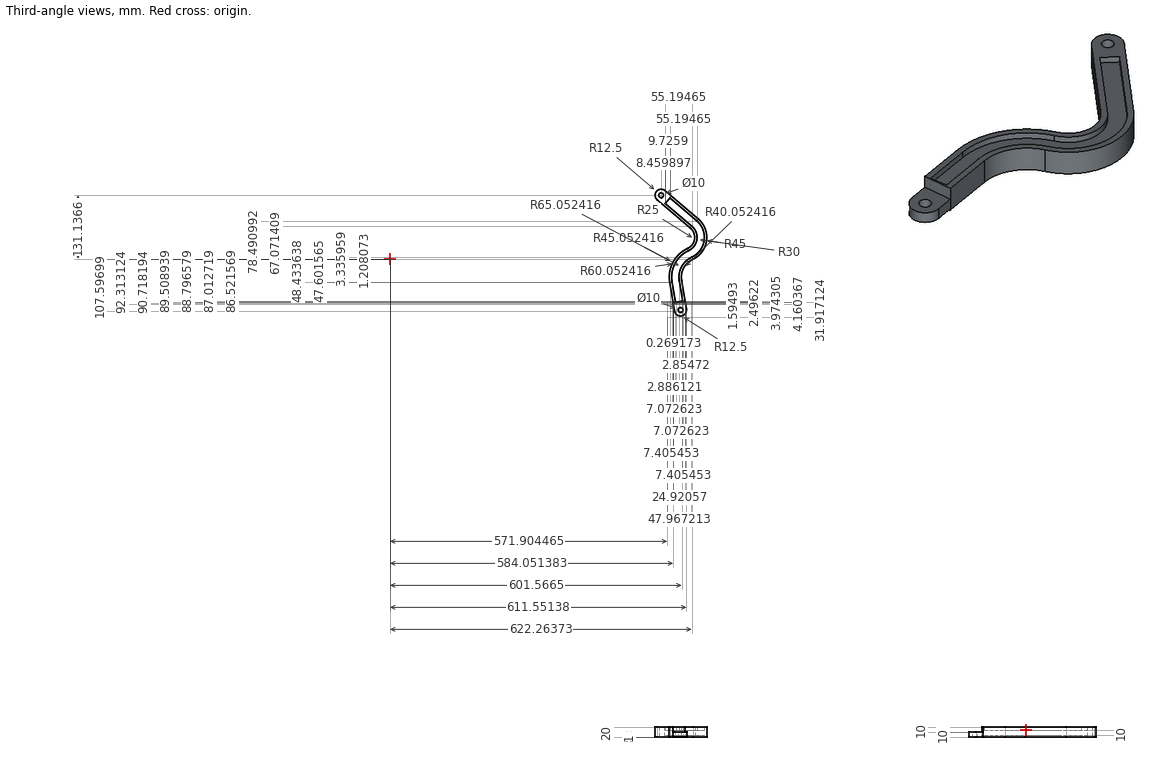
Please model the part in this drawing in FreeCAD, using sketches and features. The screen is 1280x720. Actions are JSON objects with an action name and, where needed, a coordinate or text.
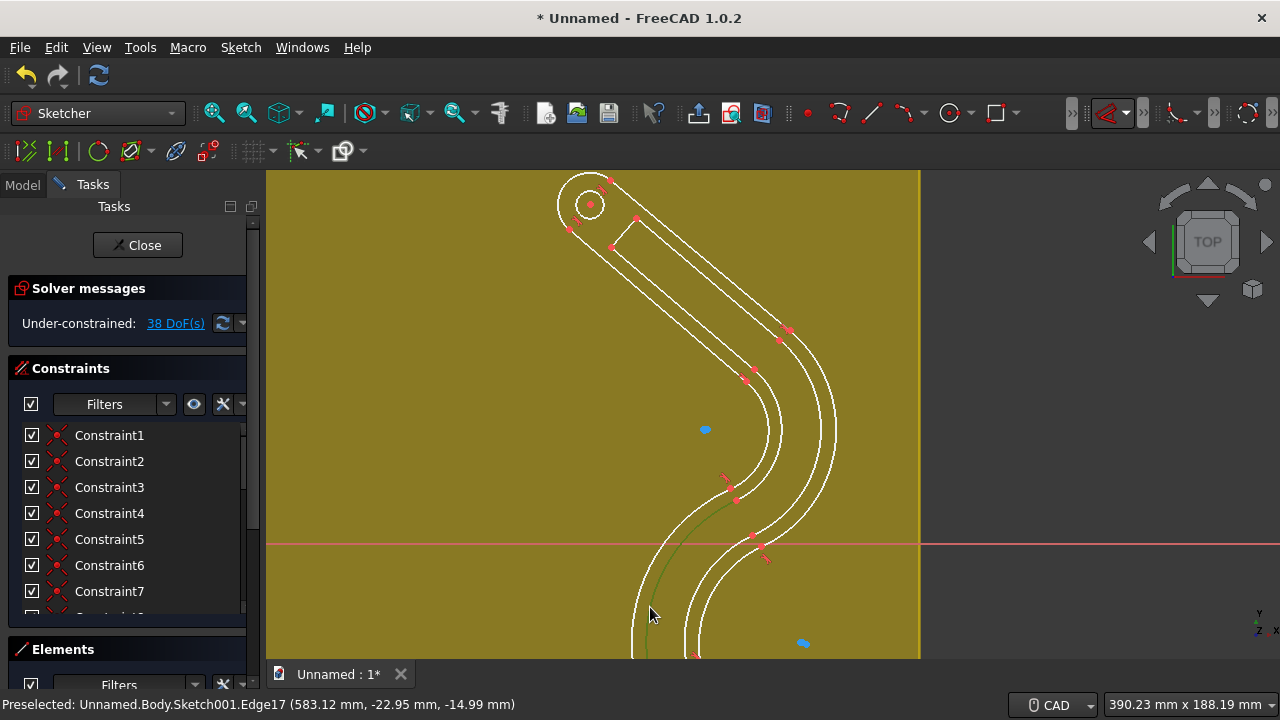
{"action": "left_click", "coordinate": [771, 469]}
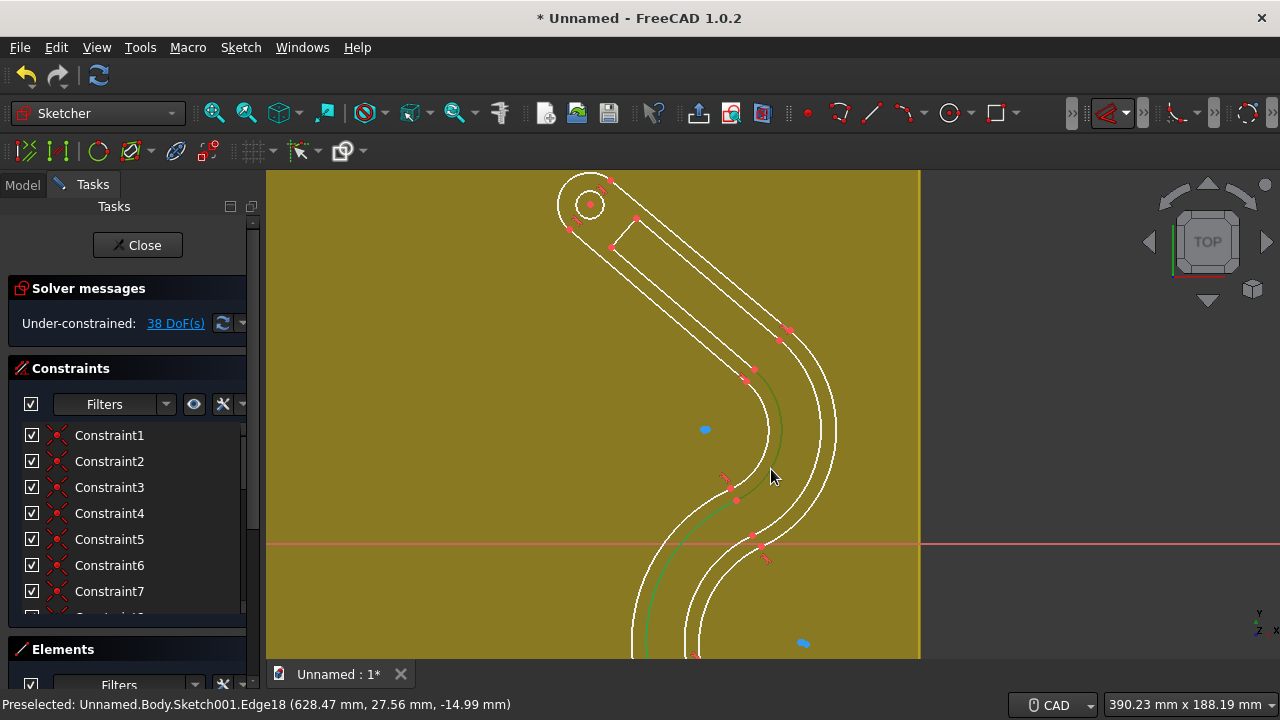
{"action": "key", "text": "t"}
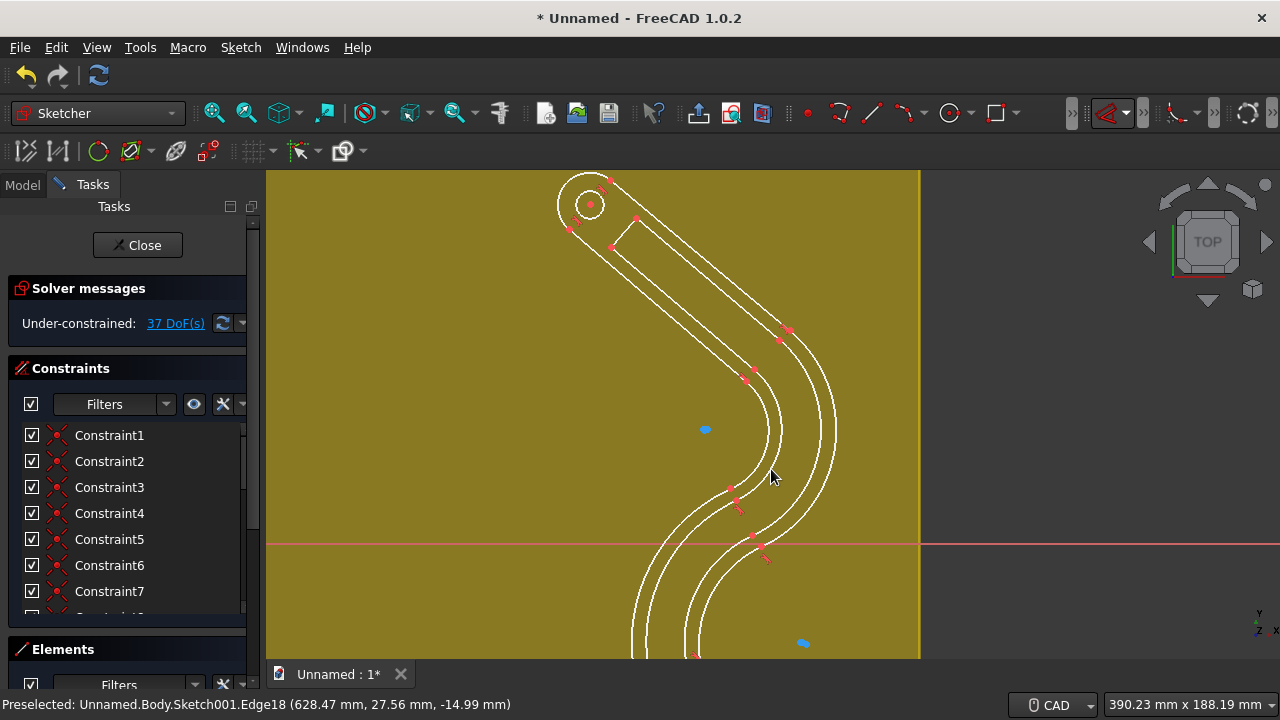
{"action": "left_click", "coordinate": [804, 489]}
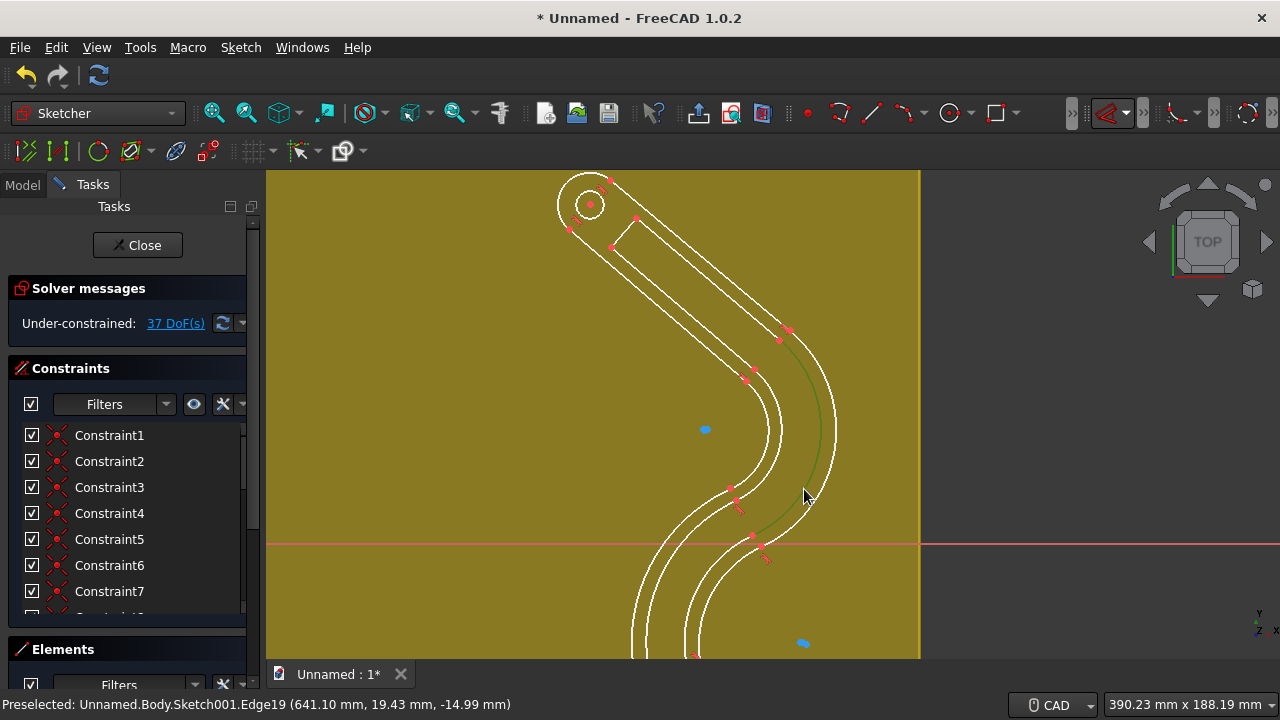
{"action": "left_click", "coordinate": [716, 562]}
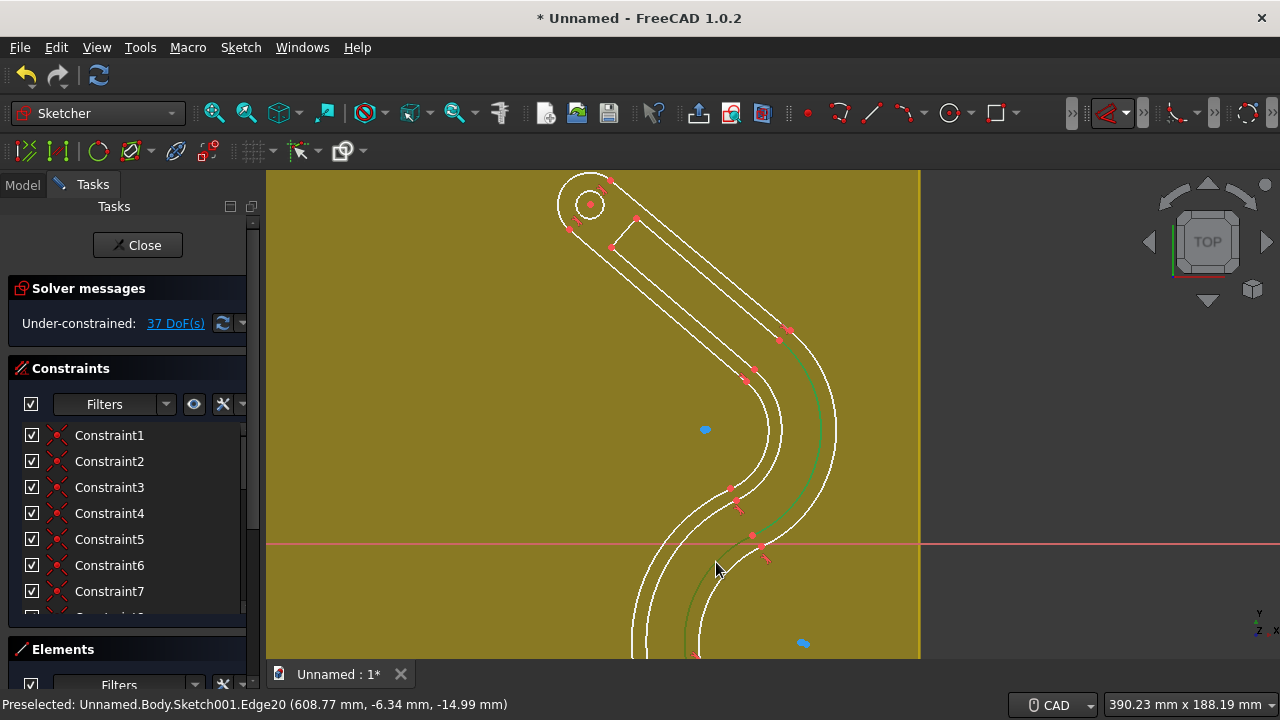
{"action": "key", "text": "t"}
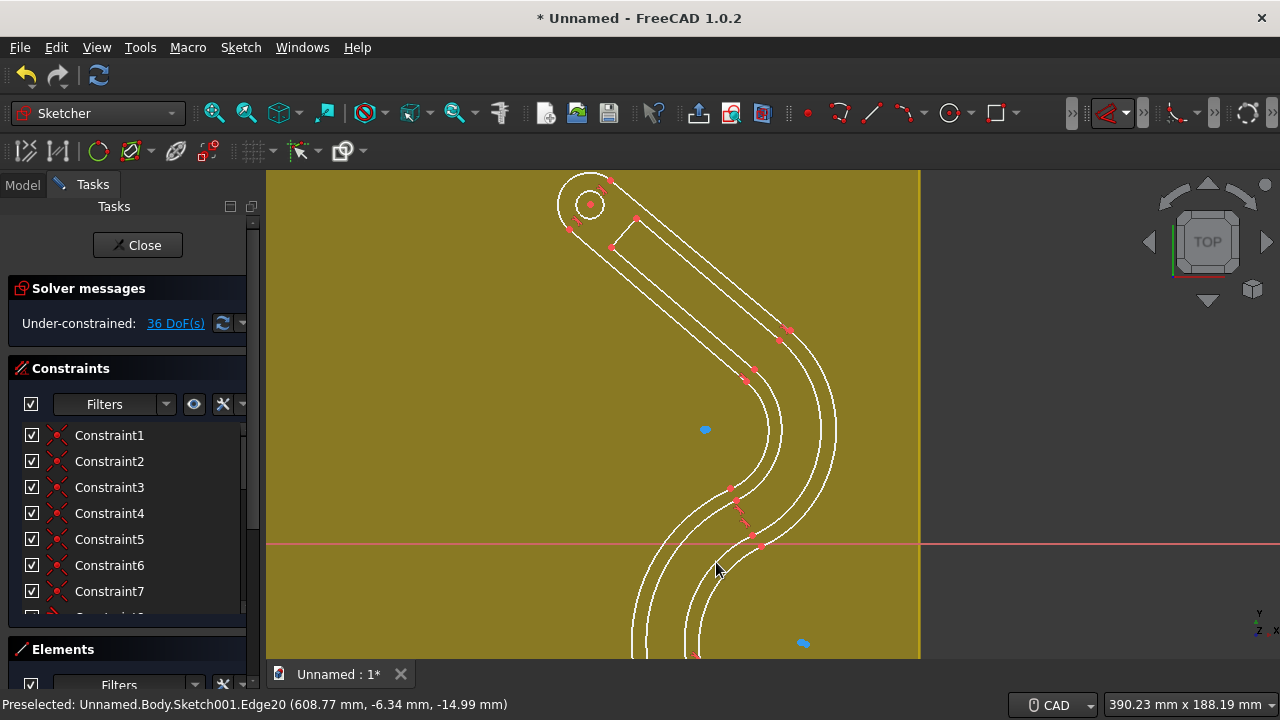
{"action": "left_click", "coordinate": [677, 528]}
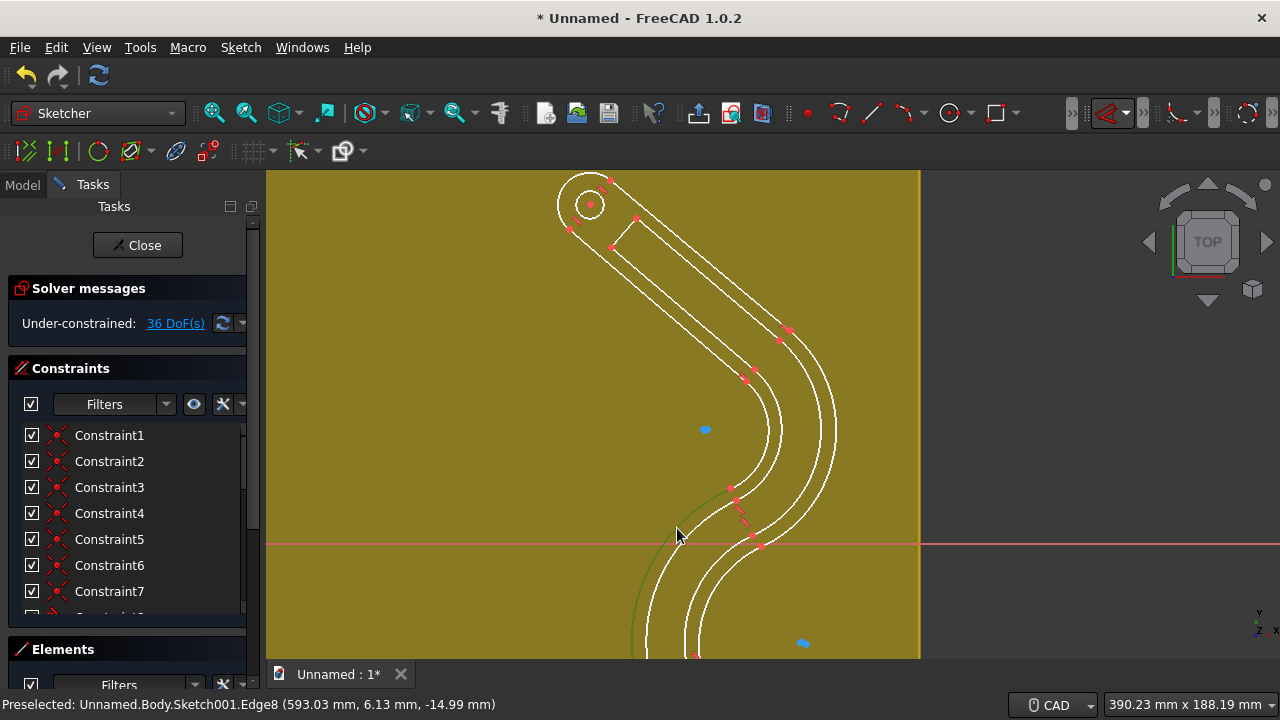
{"action": "left_click", "coordinate": [728, 571]}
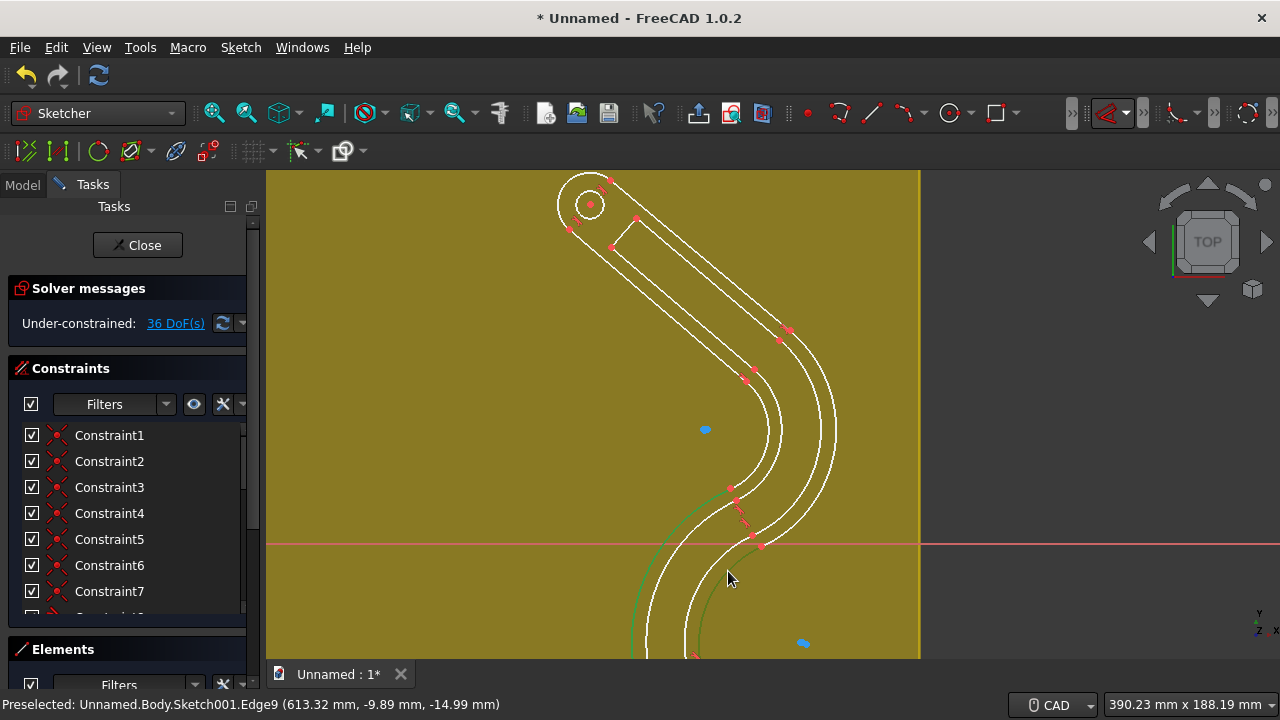
{"action": "key", "text": "c"}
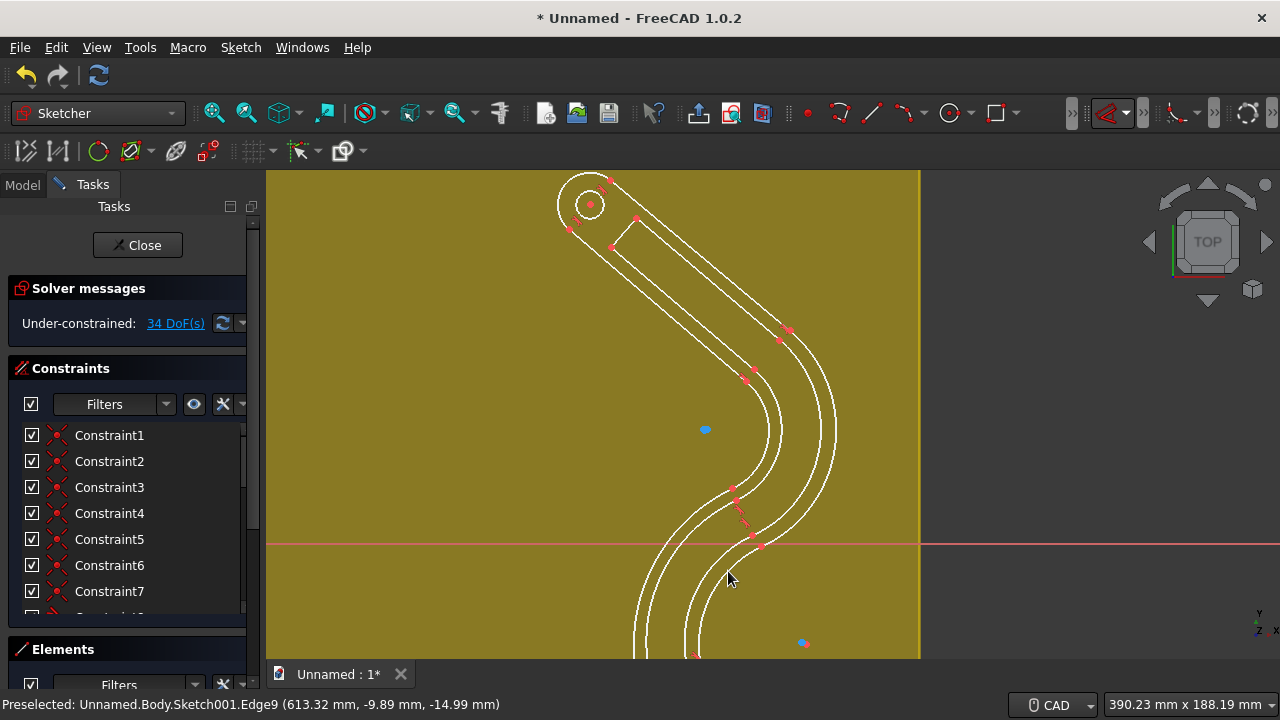
{"action": "left_click", "coordinate": [760, 463]}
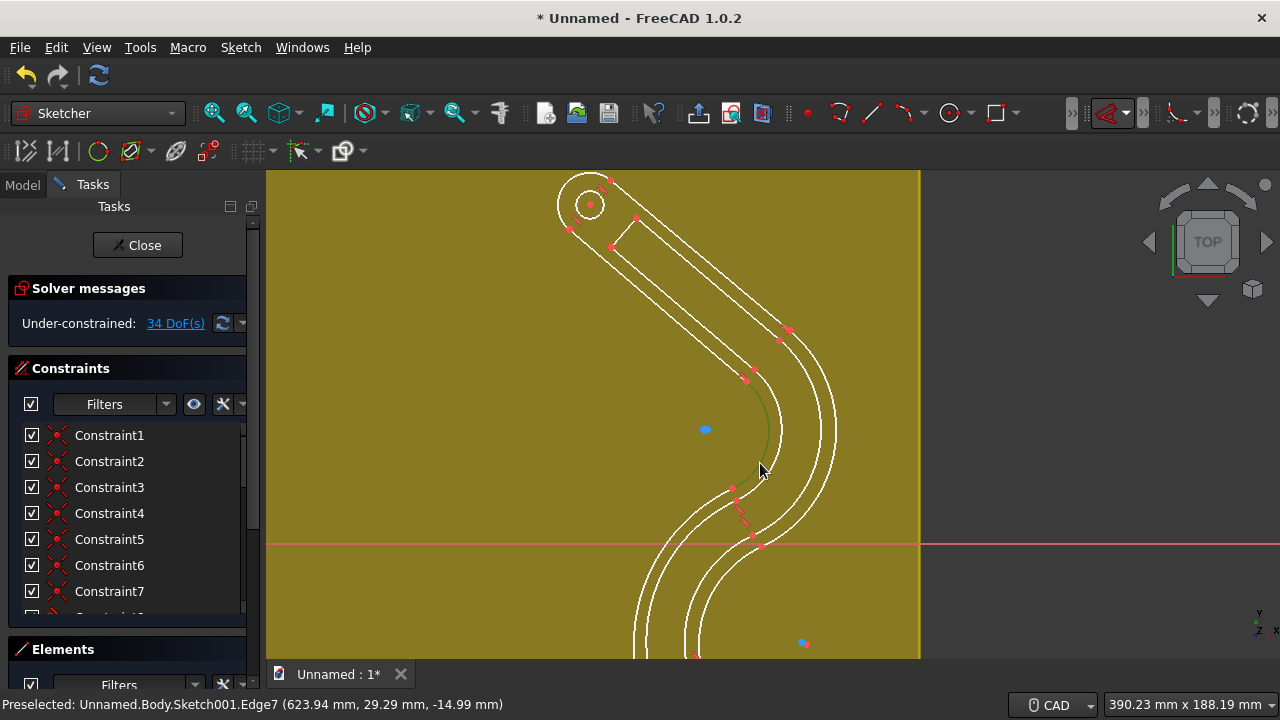
{"action": "left_click", "coordinate": [818, 496]}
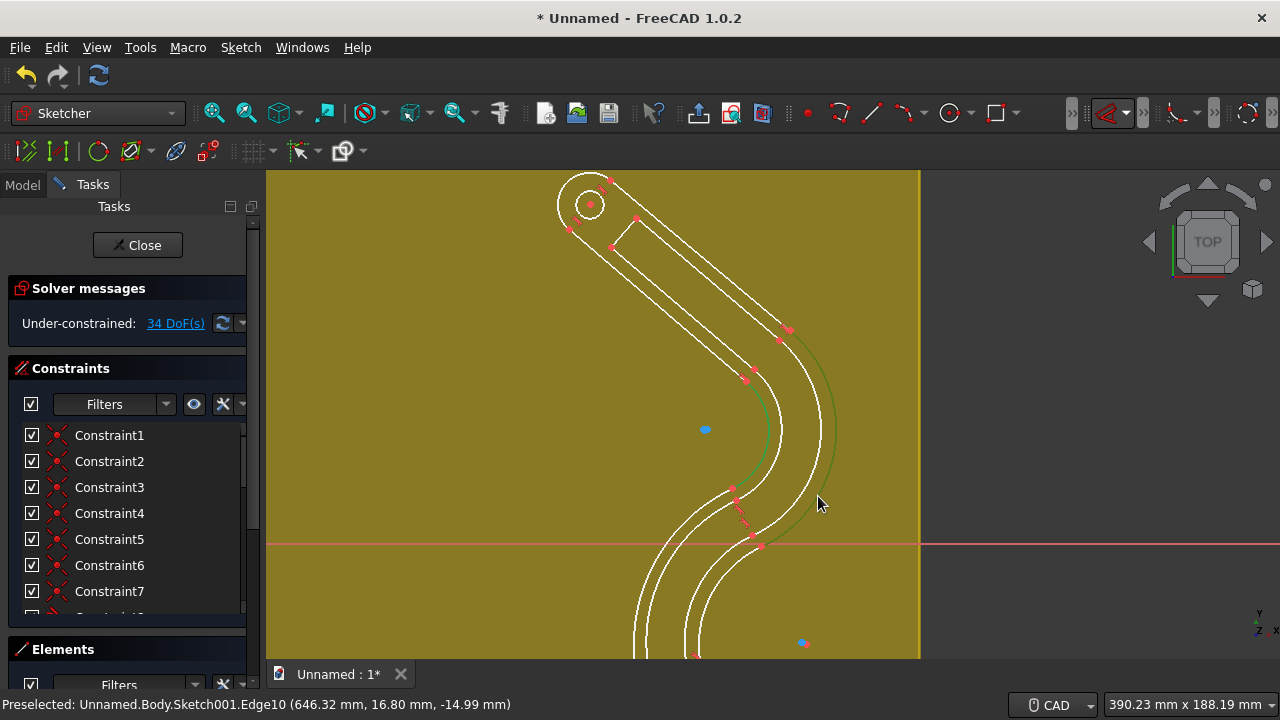
{"action": "key", "text": "c"}